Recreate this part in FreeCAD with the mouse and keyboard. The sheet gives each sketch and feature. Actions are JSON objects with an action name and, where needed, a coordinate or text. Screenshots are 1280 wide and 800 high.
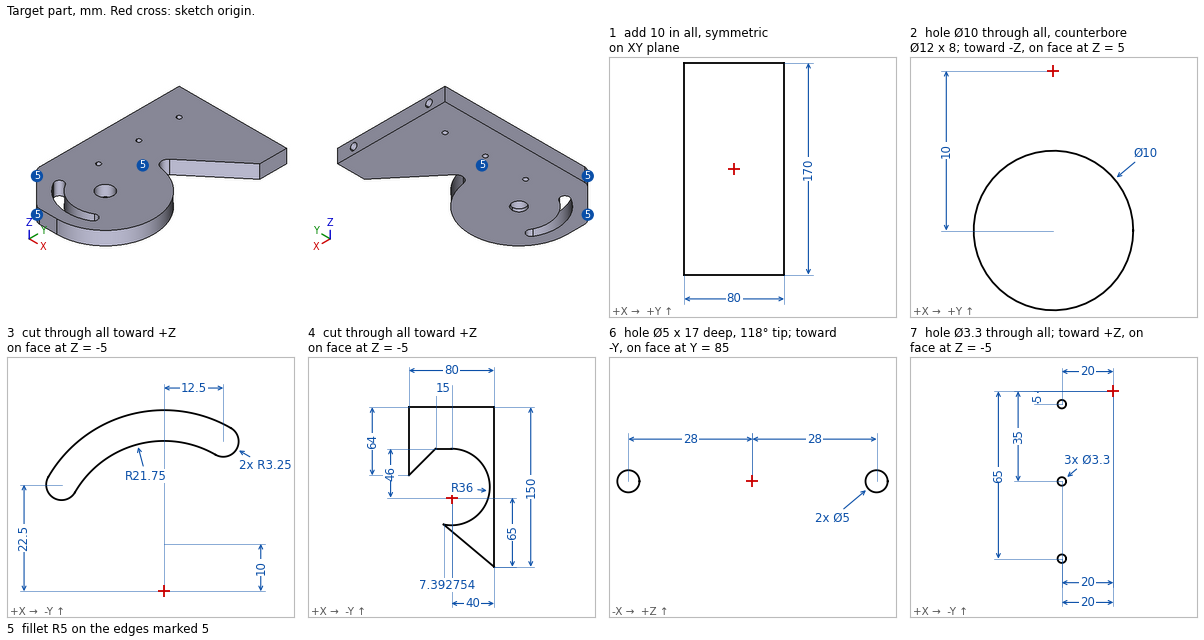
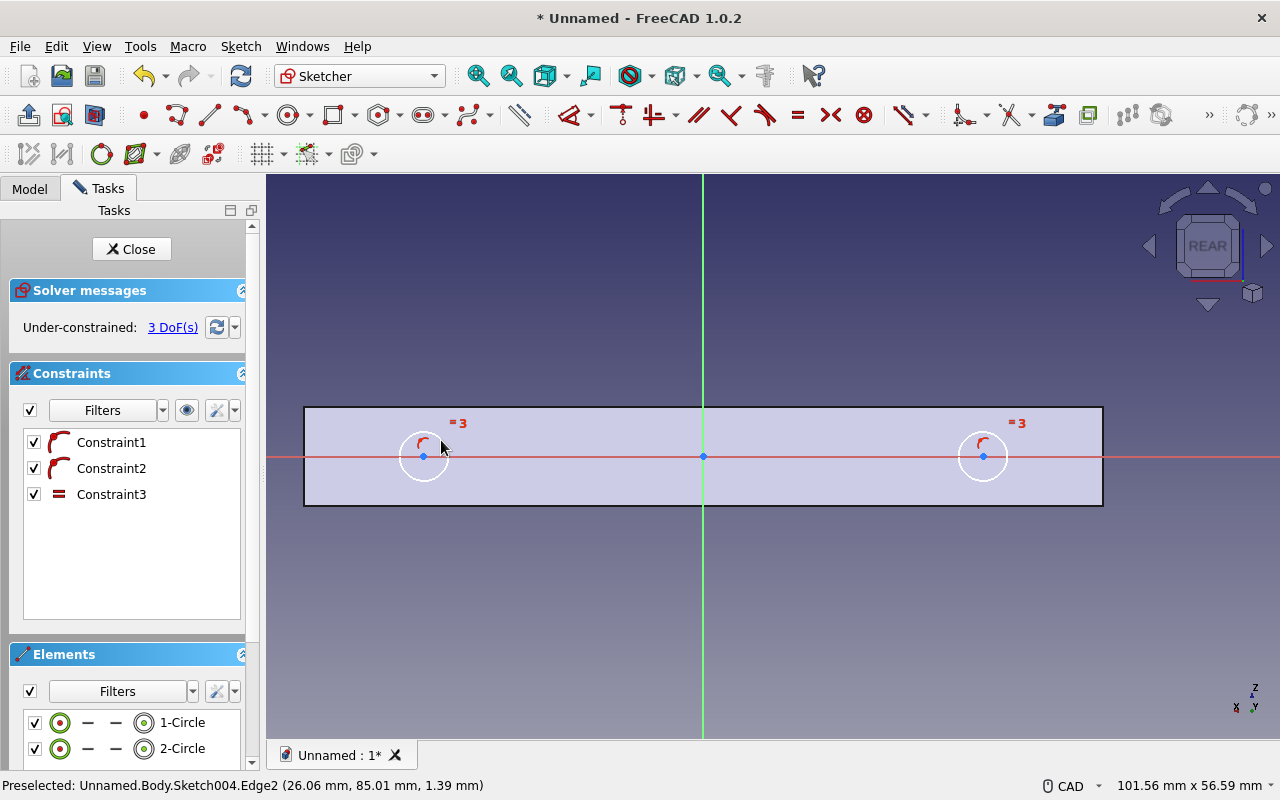
{"action": "key", "text": "d"}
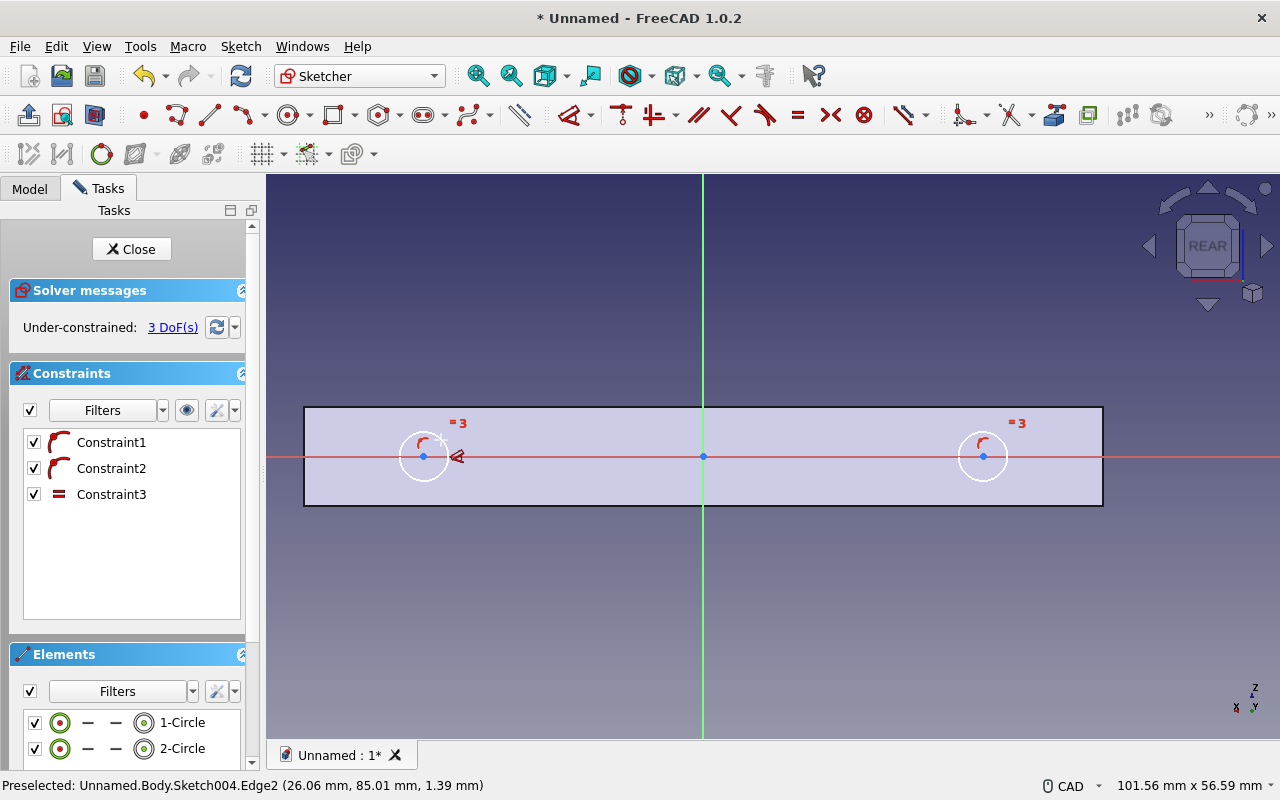
{"action": "left_click", "coordinate": [1000, 439]}
{"action": "left_click", "coordinate": [1022, 416]}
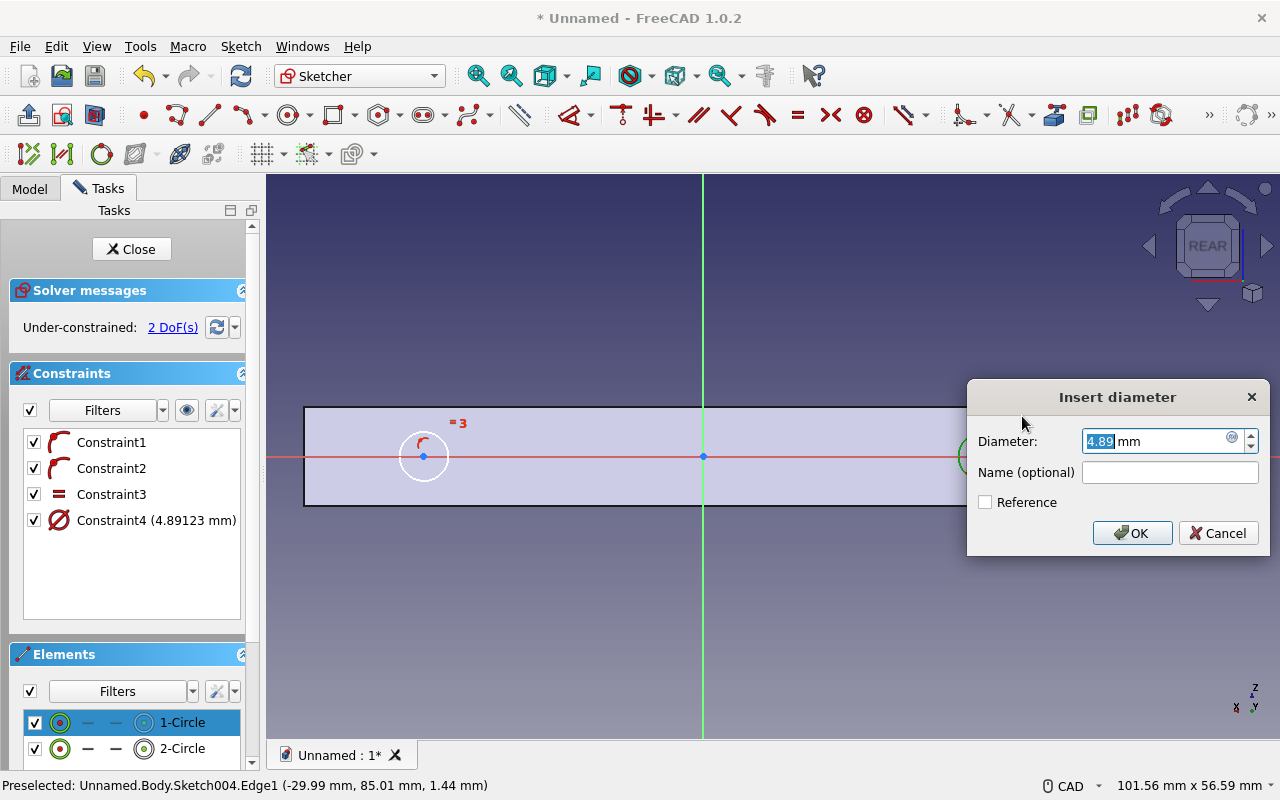
{"action": "type", "text": "5"}
{"action": "key", "text": "Return"}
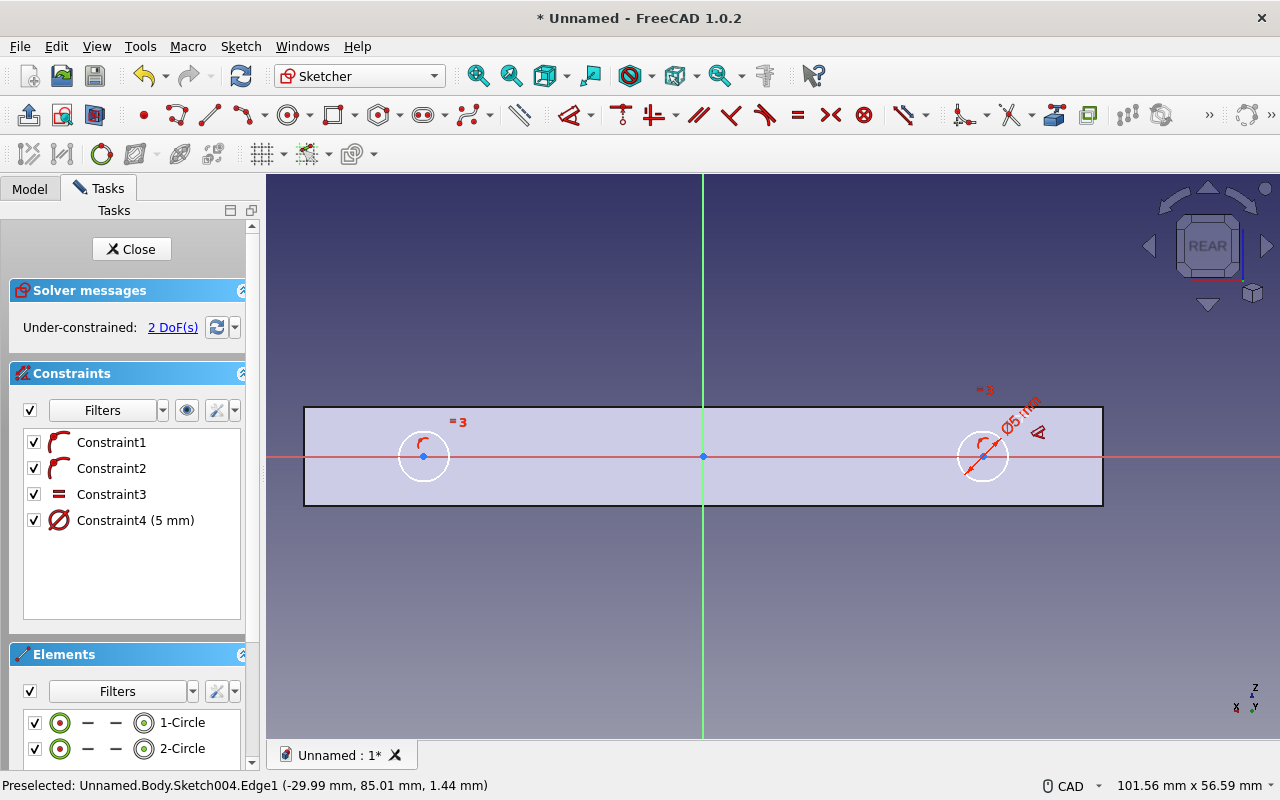
{"action": "left_click", "coordinate": [983, 456]}
{"action": "left_click", "coordinate": [843, 490]}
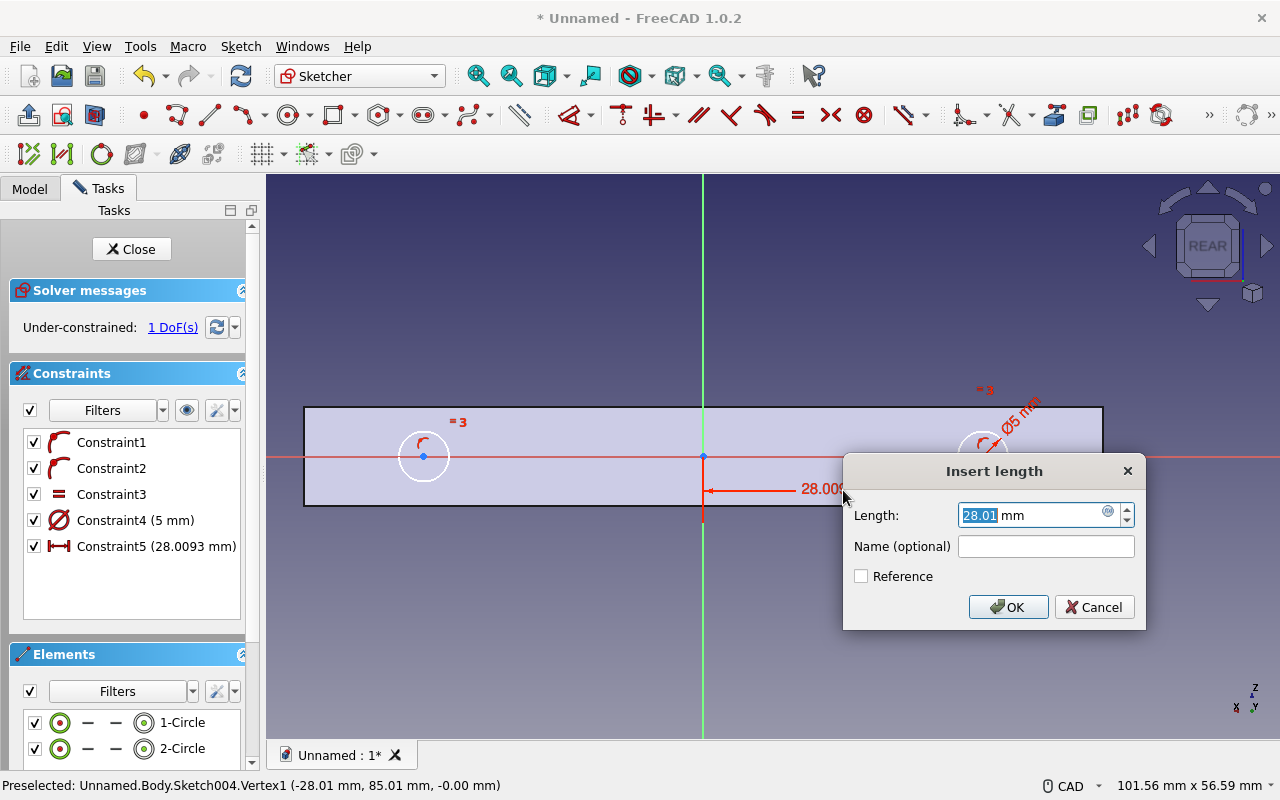
{"action": "type", "text": "28"}
{"action": "key", "text": "Return"}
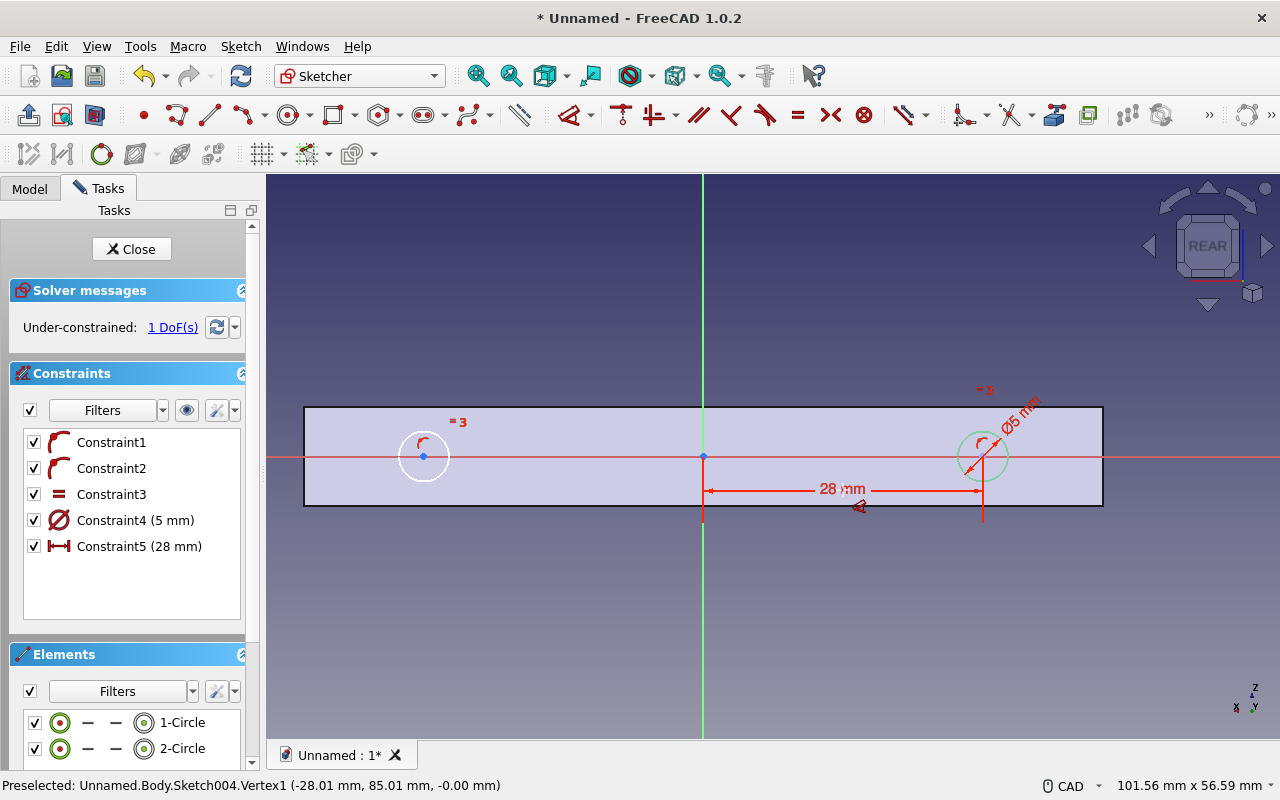
{"action": "left_click", "coordinate": [424, 456]}
{"action": "left_click", "coordinate": [564, 490]}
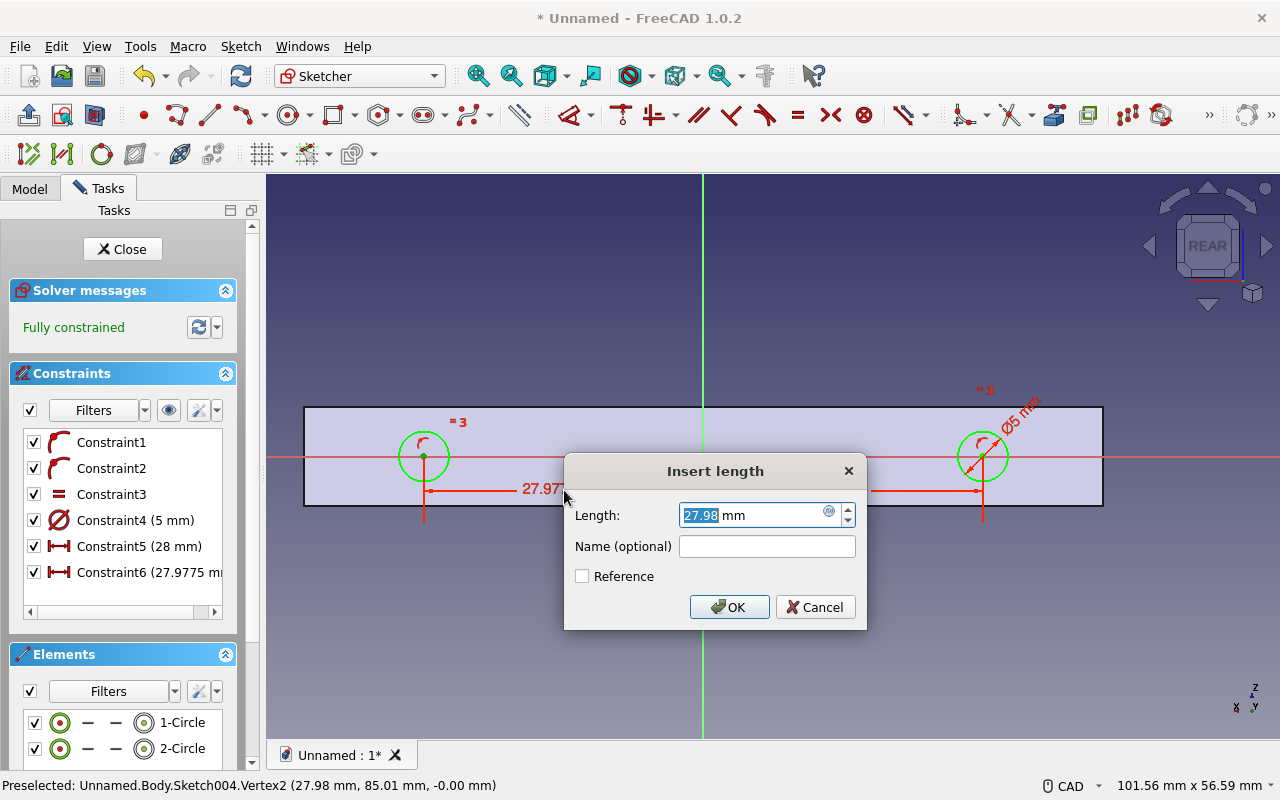
{"action": "type", "text": "28"}
{"action": "key", "text": "Return"}
{"action": "key", "text": "Escape"}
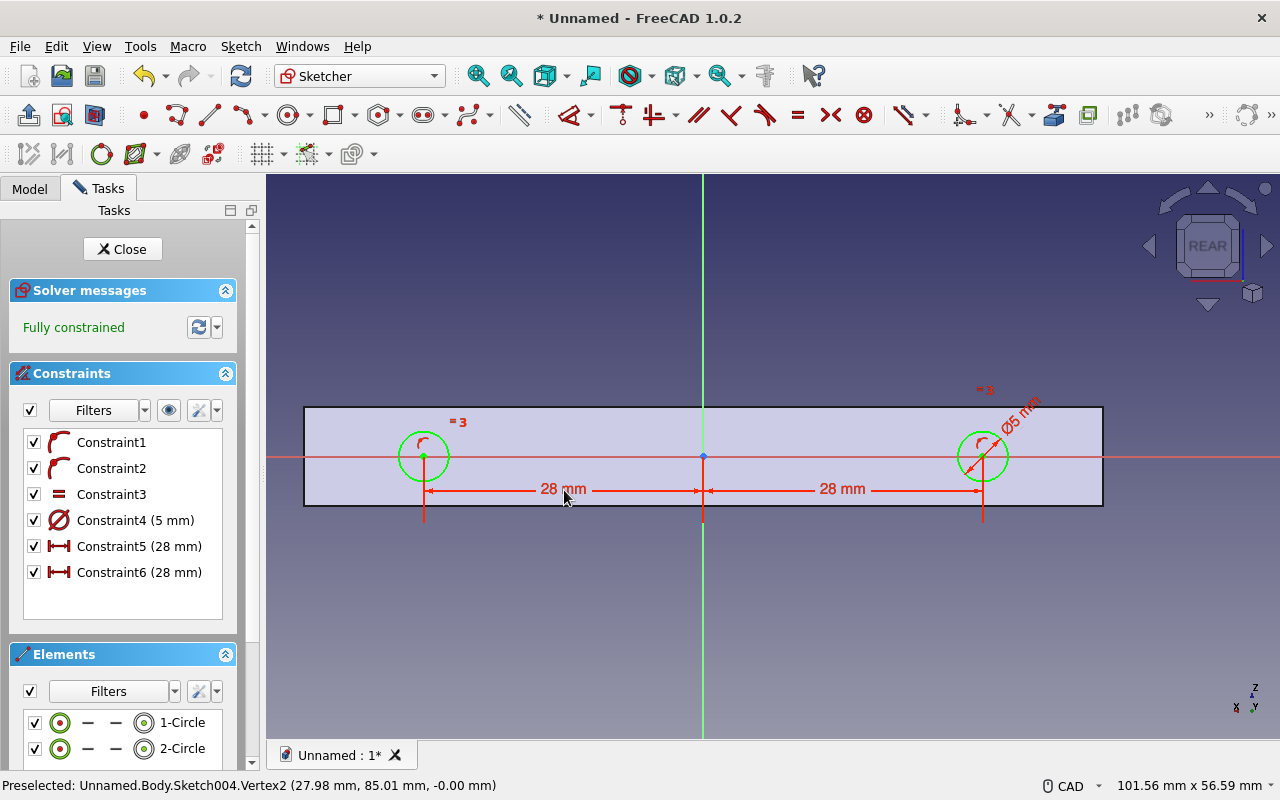
{"action": "left_click", "coordinate": [123, 249]}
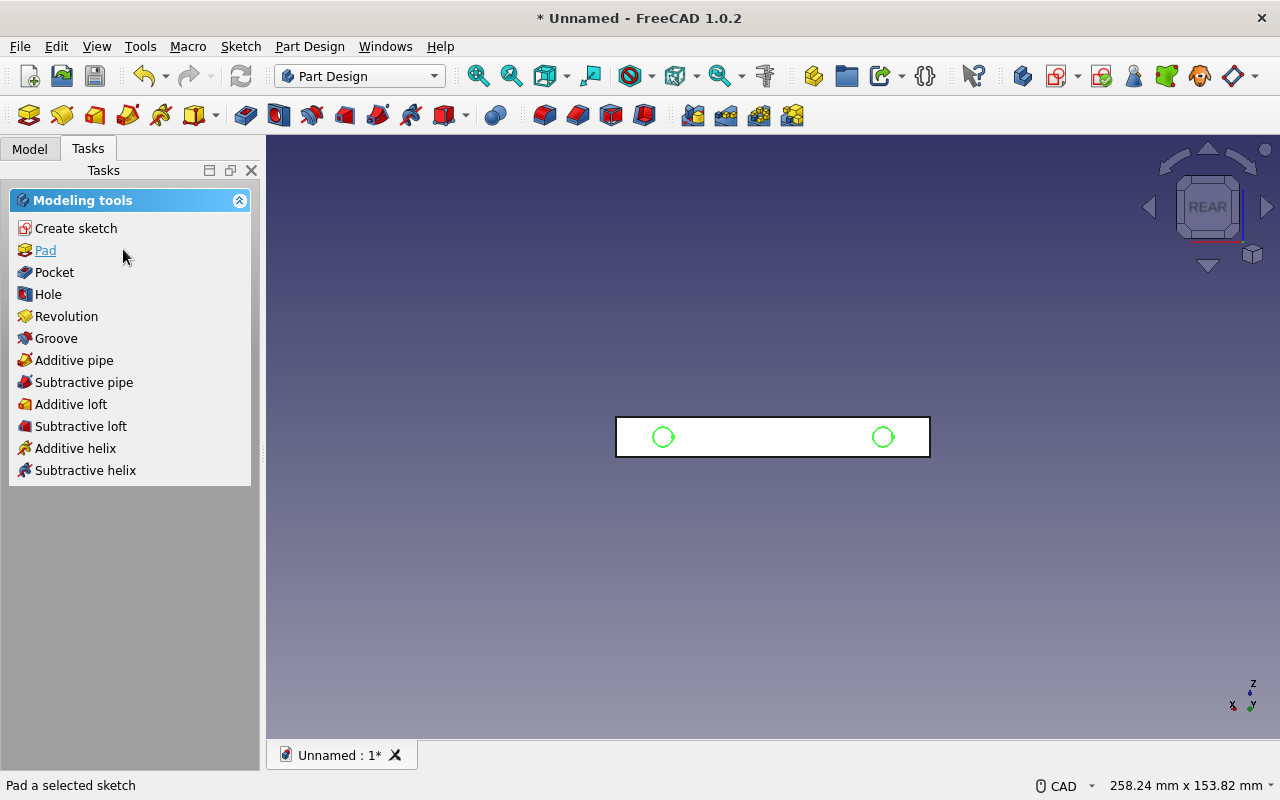
{"action": "left_click", "coordinate": [279, 116]}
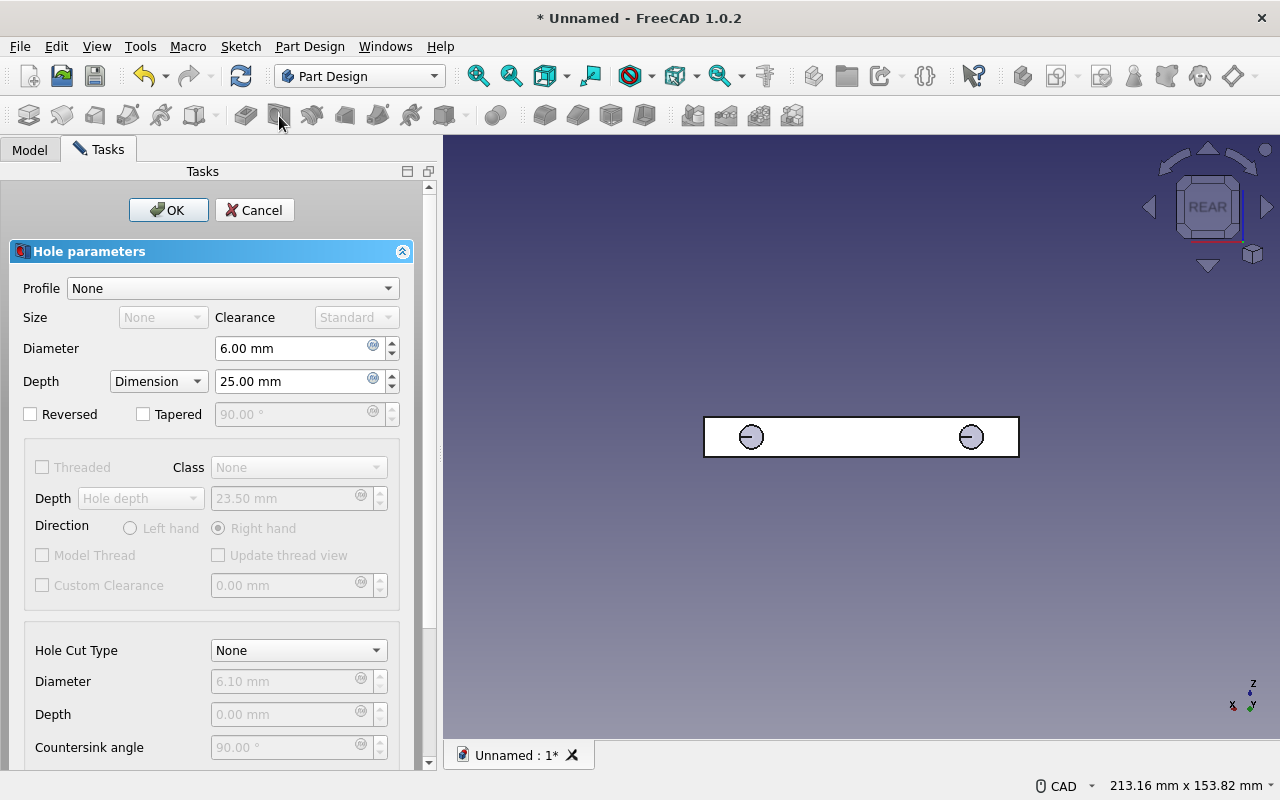
{"action": "triple_click", "coordinate": [300, 348]}